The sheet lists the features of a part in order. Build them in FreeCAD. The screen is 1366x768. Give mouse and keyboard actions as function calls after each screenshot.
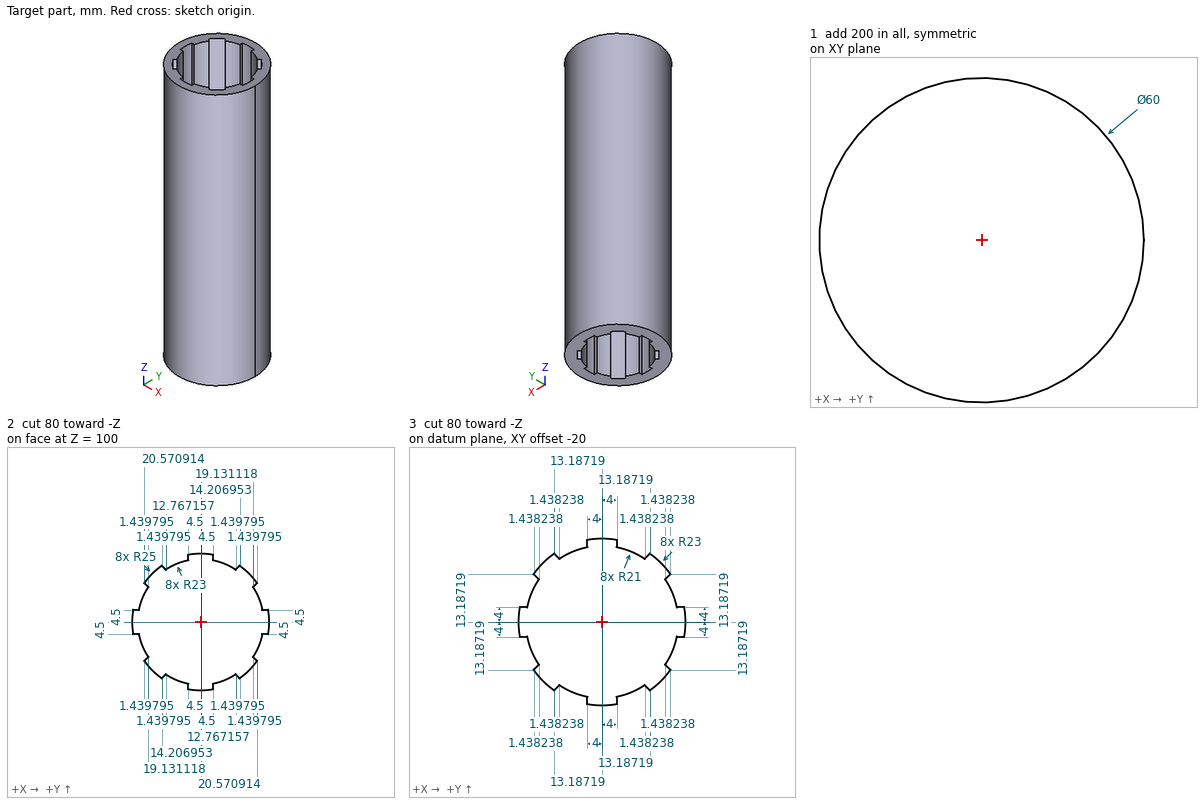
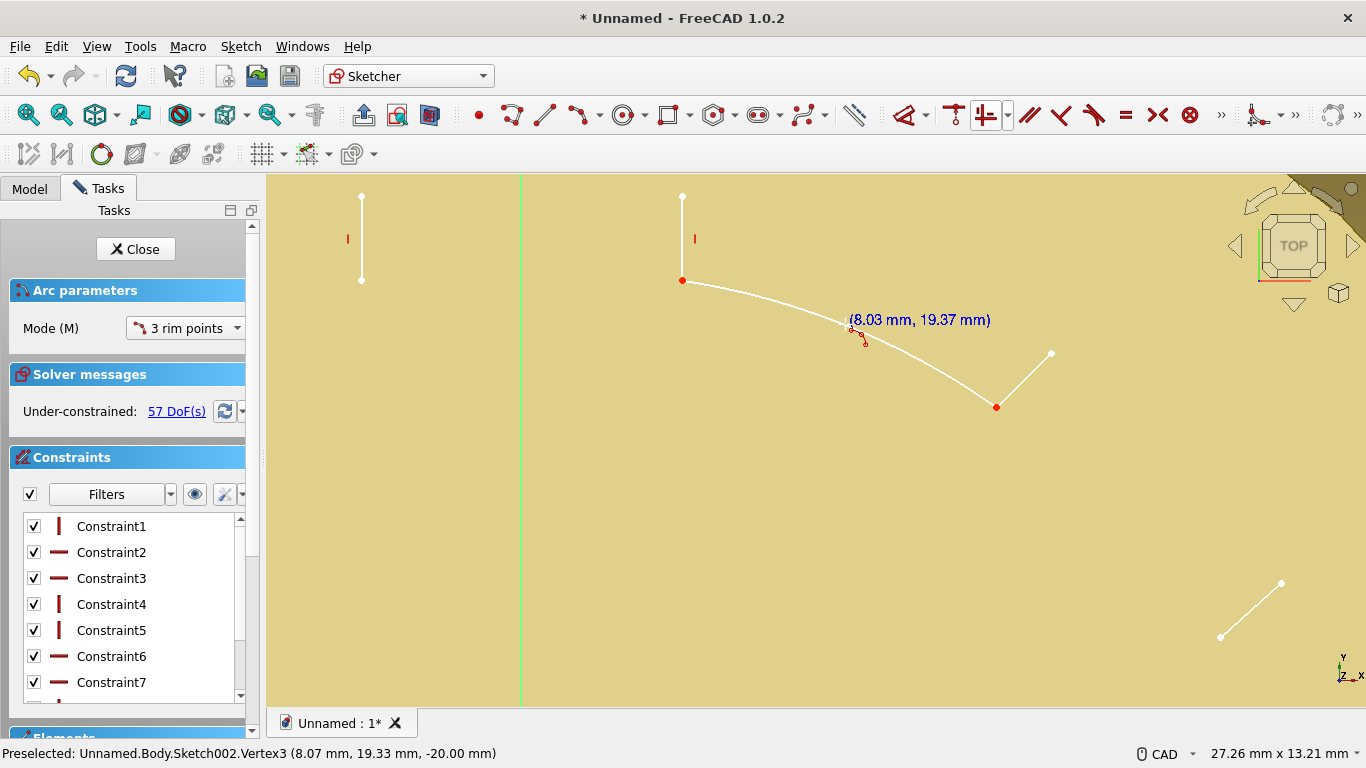
click(1051, 353)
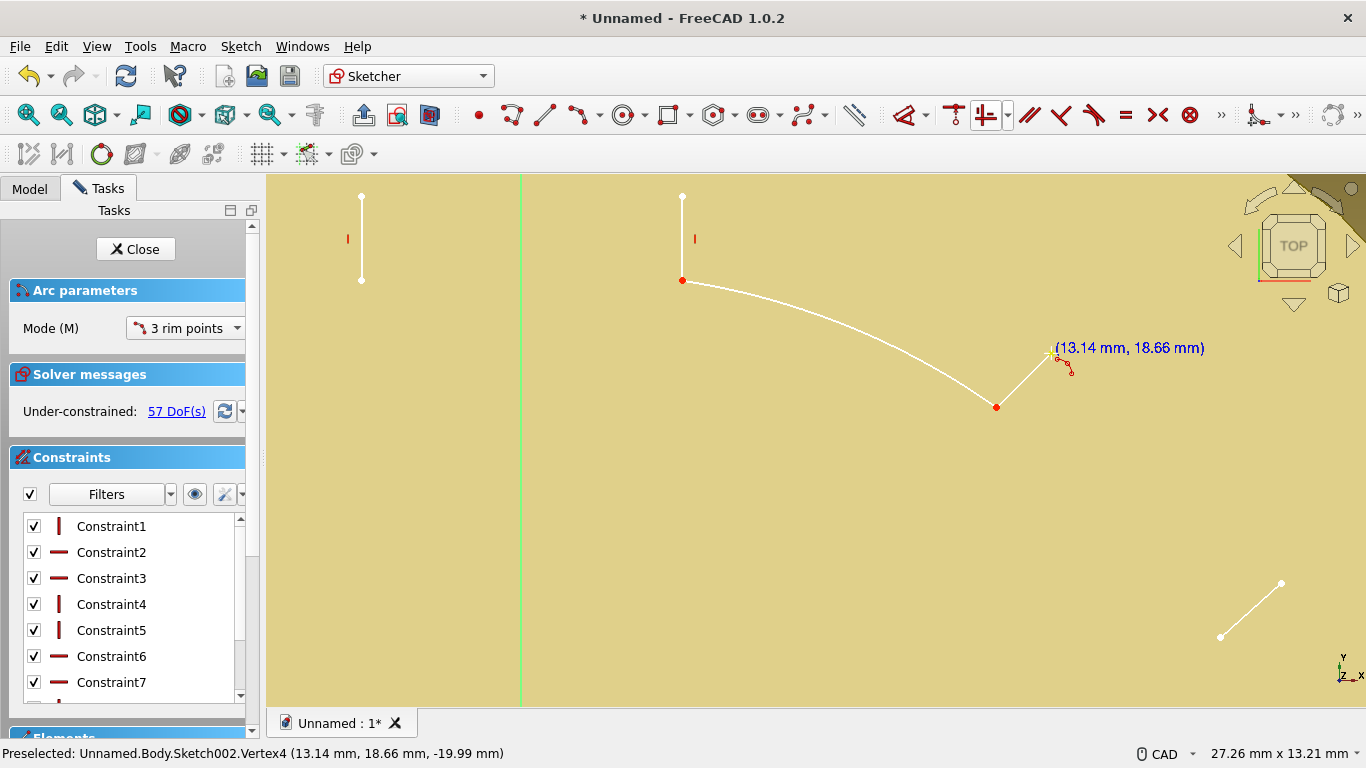
scroll(792, 309, down, 9)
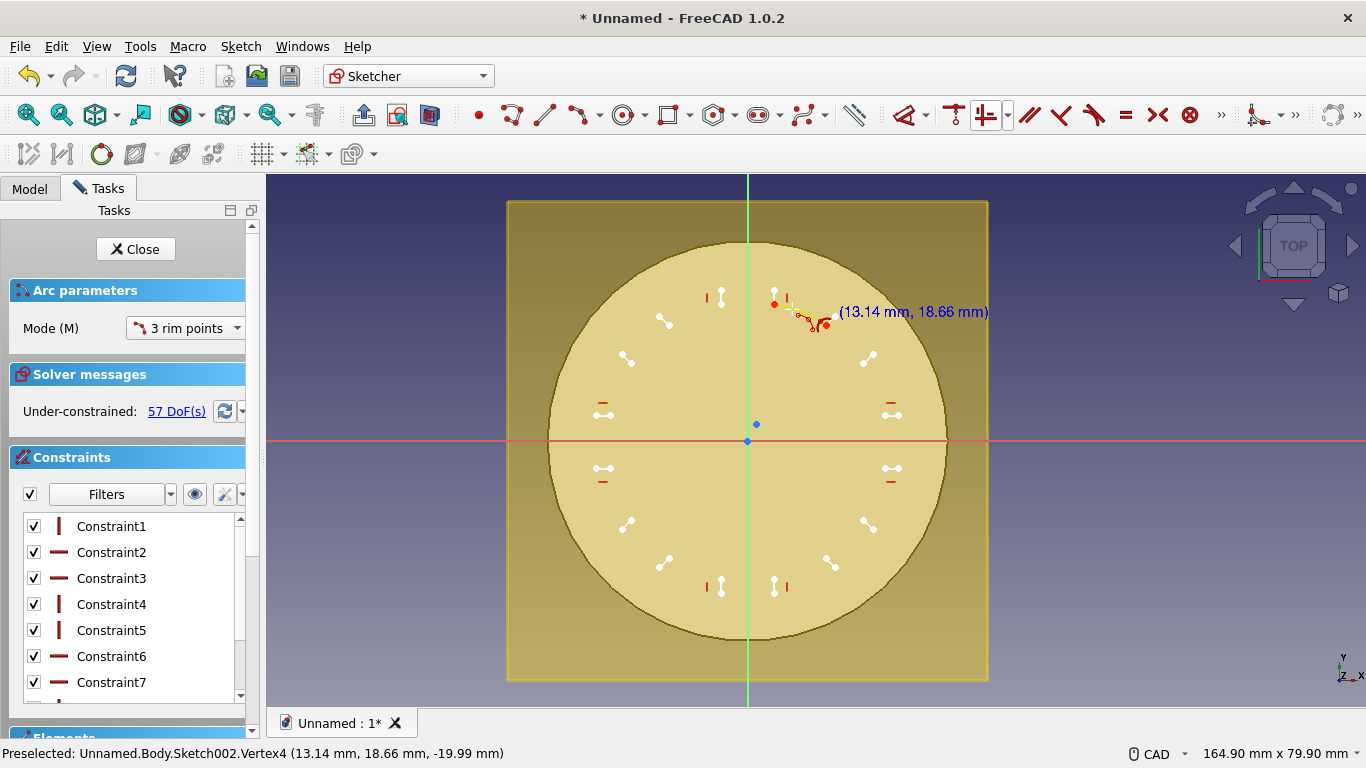
scroll(873, 353, up, 5)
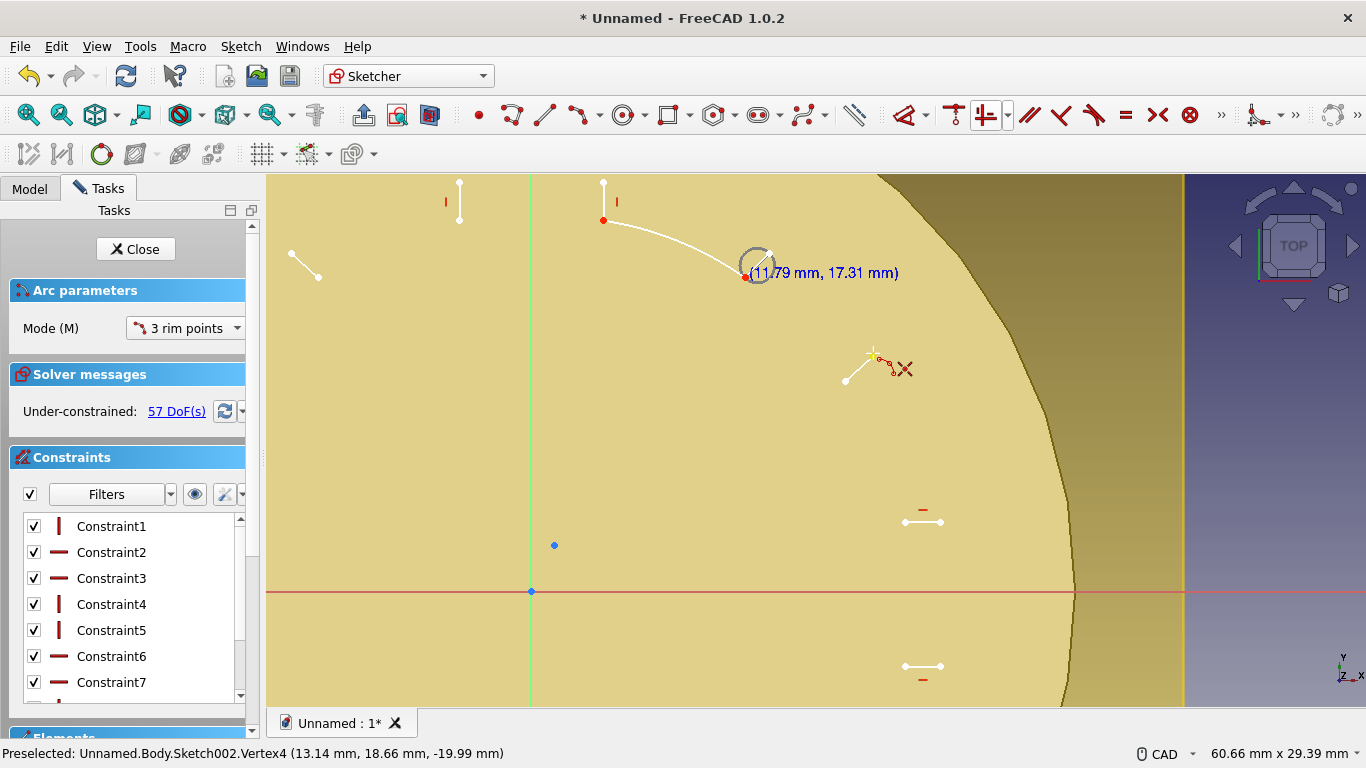
click(873, 357)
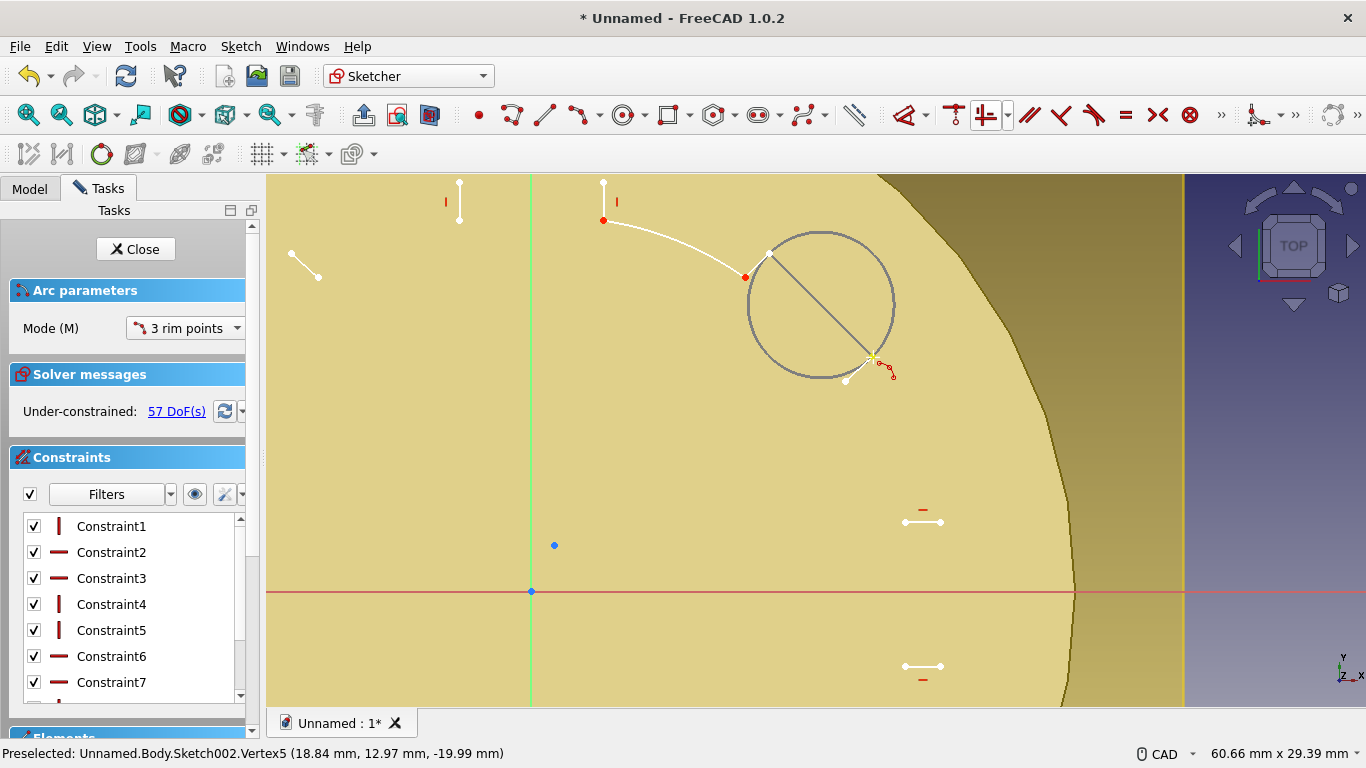
scroll(826, 297, up, 5)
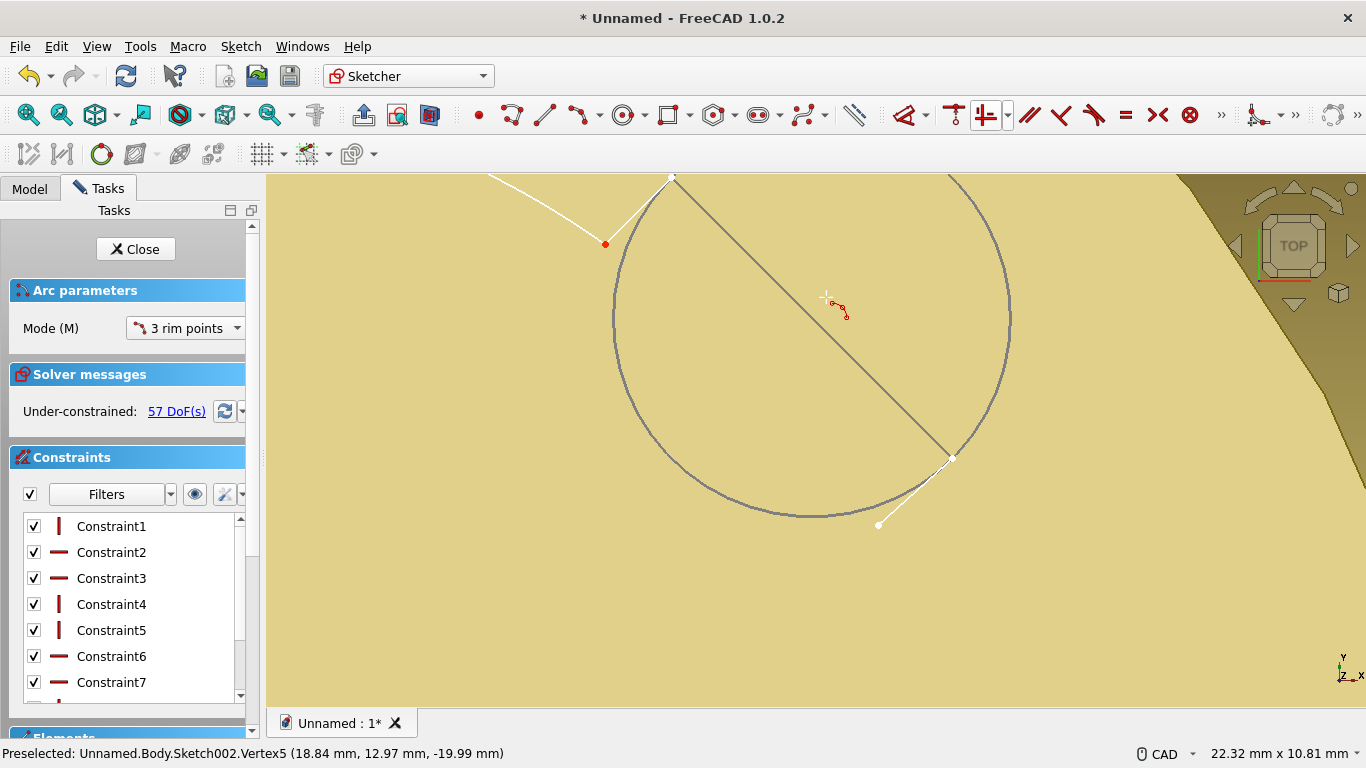
click(825, 296)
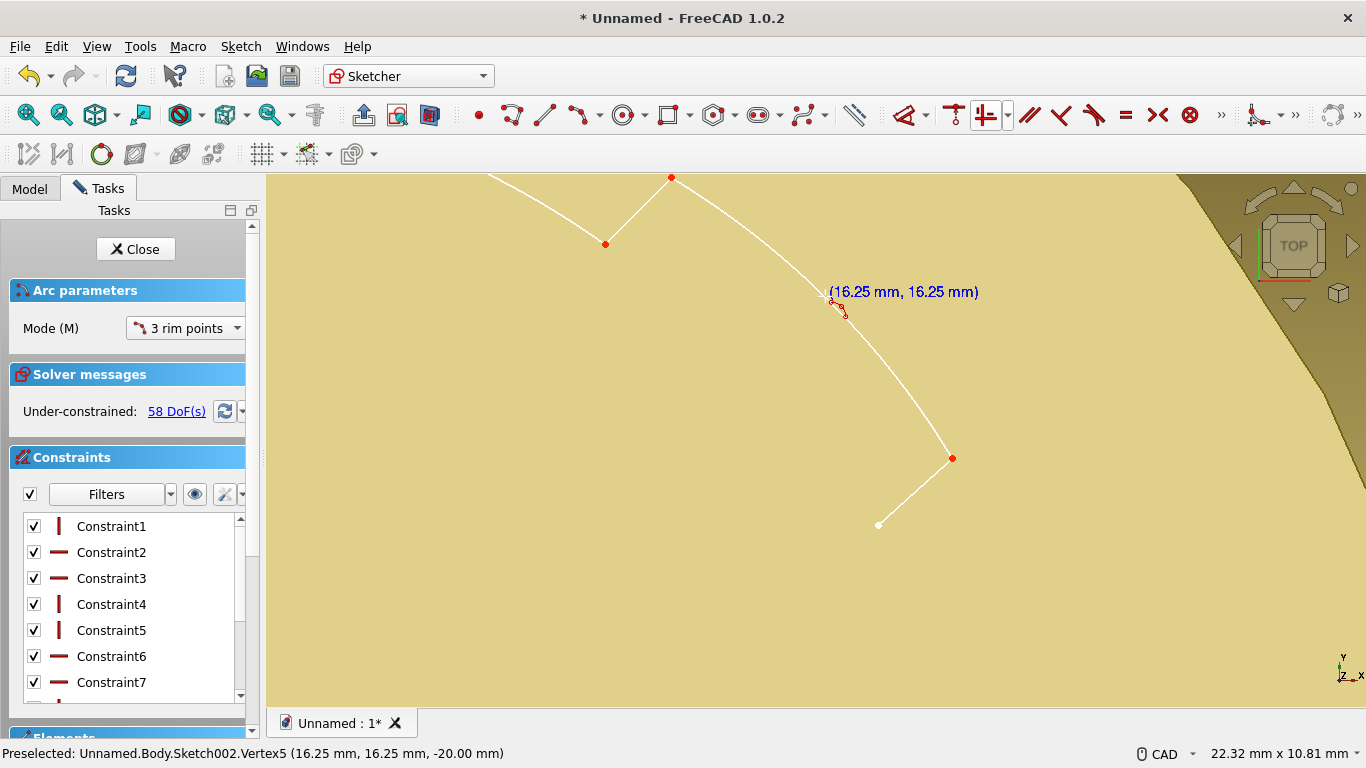
scroll(861, 338, down, 10)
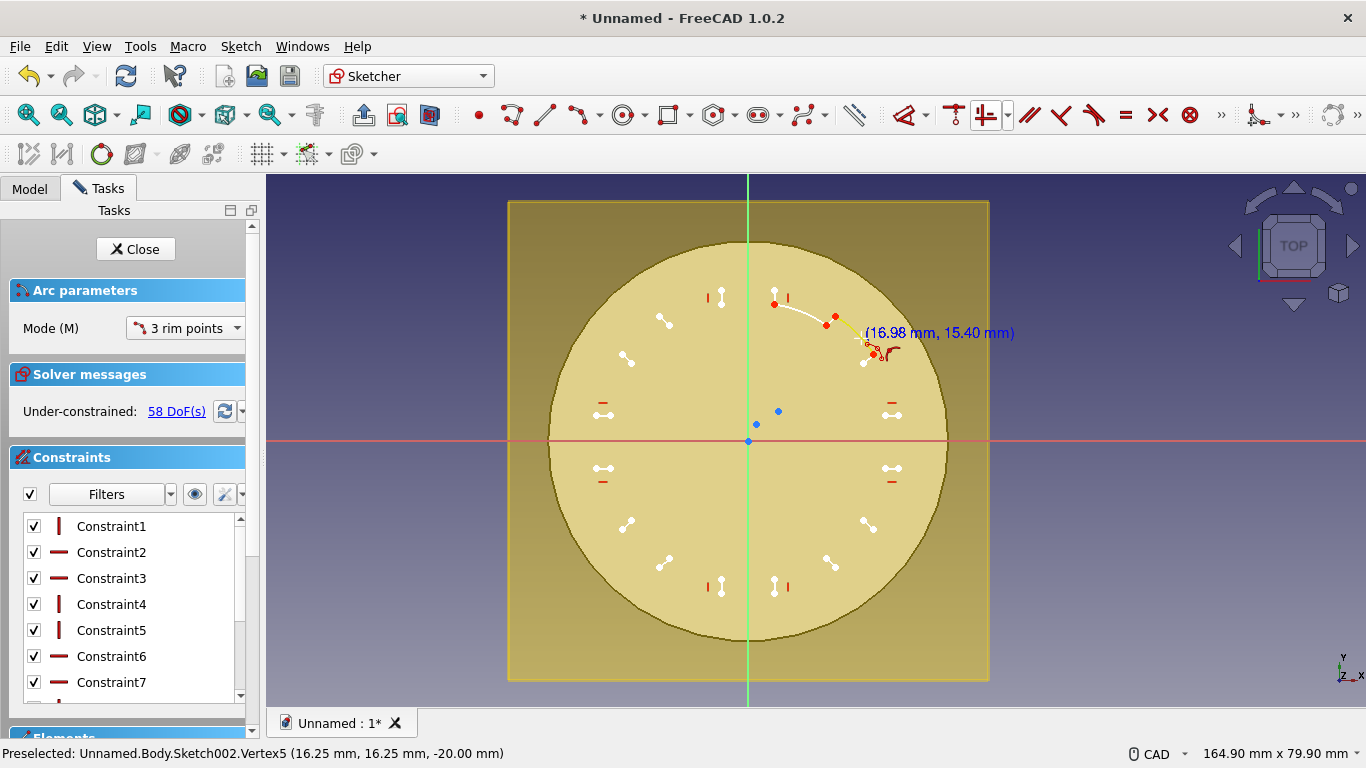
scroll(864, 363, up, 5)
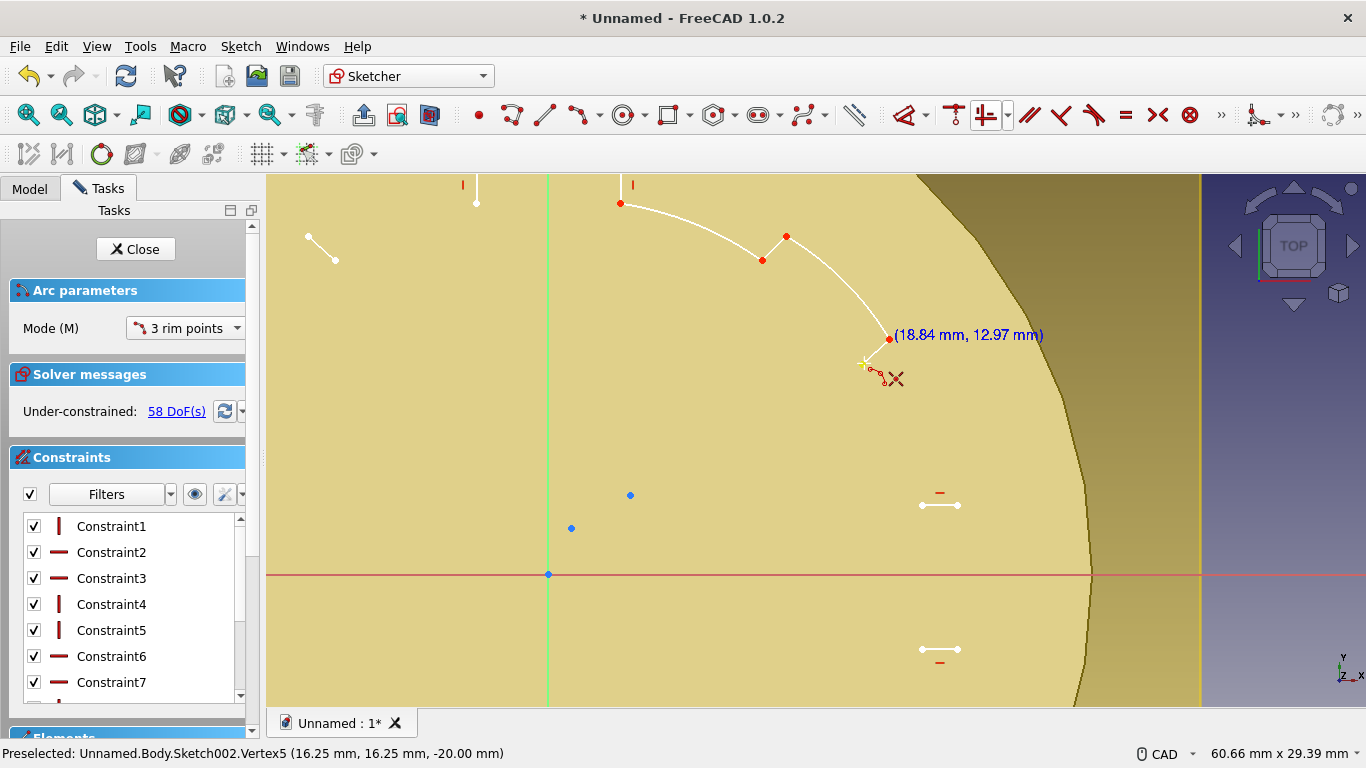
click(863, 364)
click(922, 505)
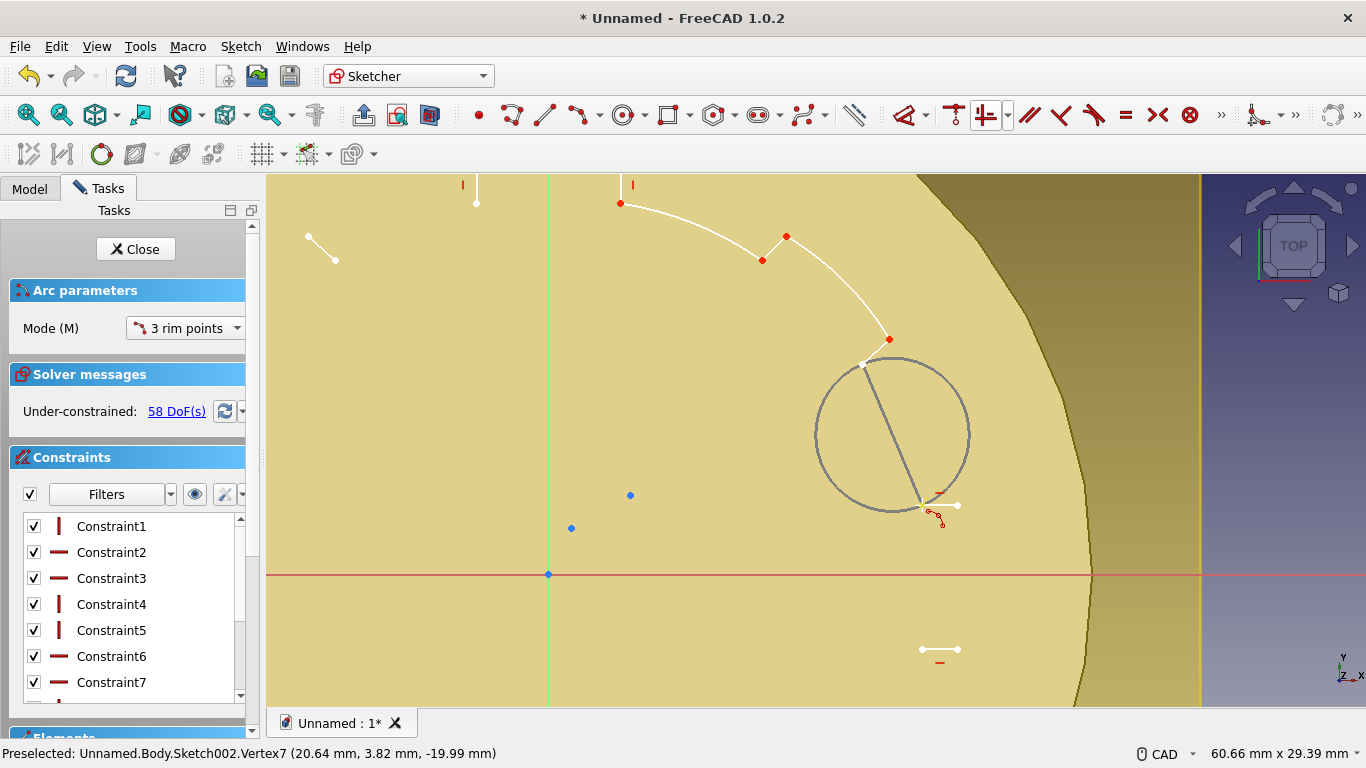
scroll(900, 429, up, 4)